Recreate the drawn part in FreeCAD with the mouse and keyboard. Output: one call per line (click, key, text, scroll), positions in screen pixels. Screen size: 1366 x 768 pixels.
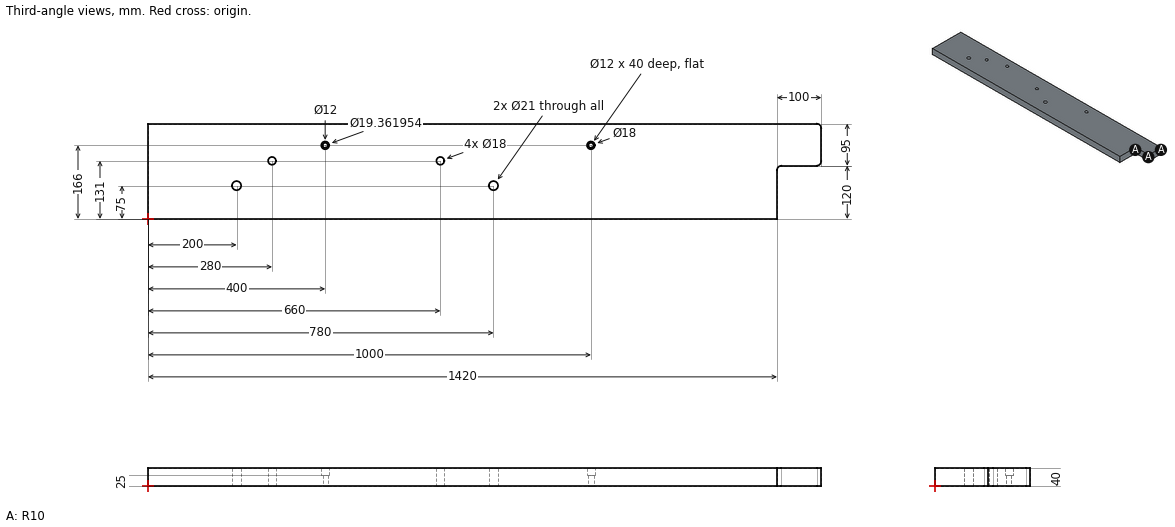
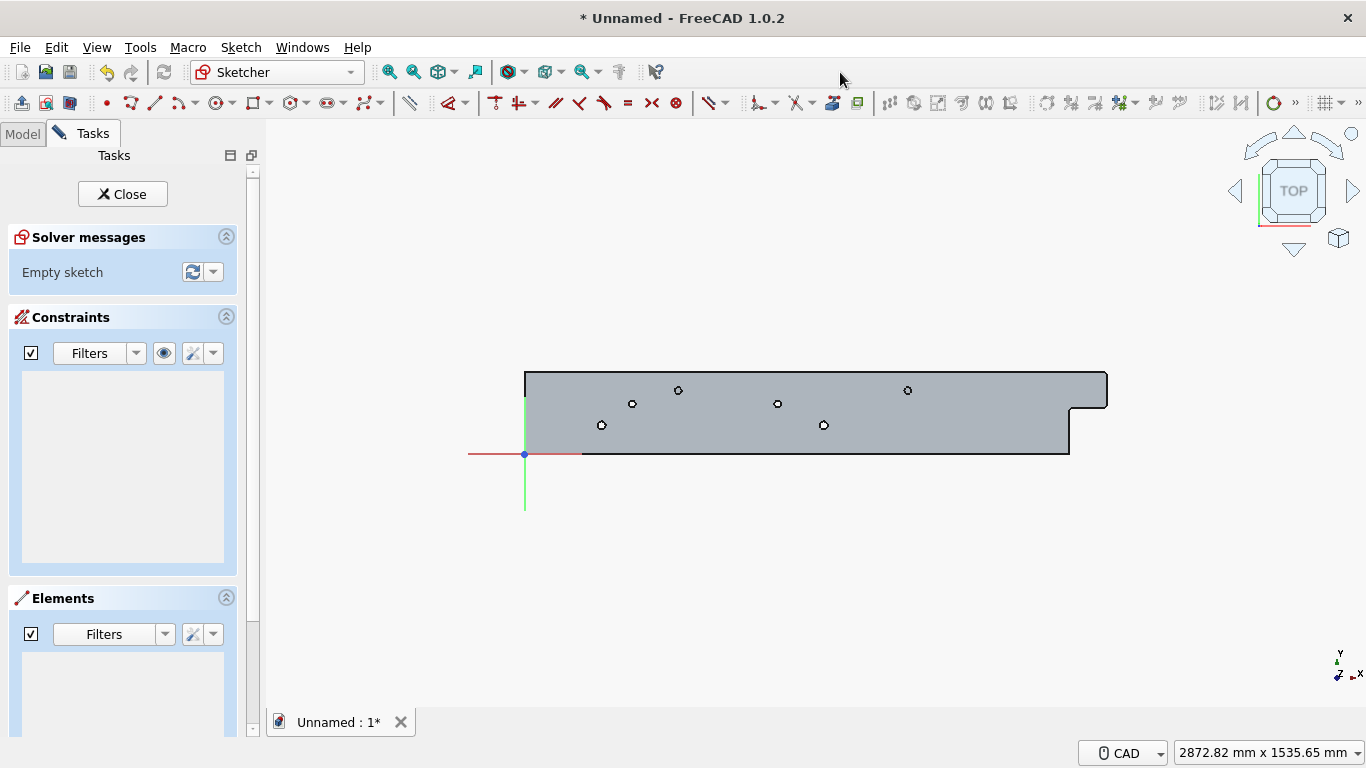
scroll(916, 389, up, 15)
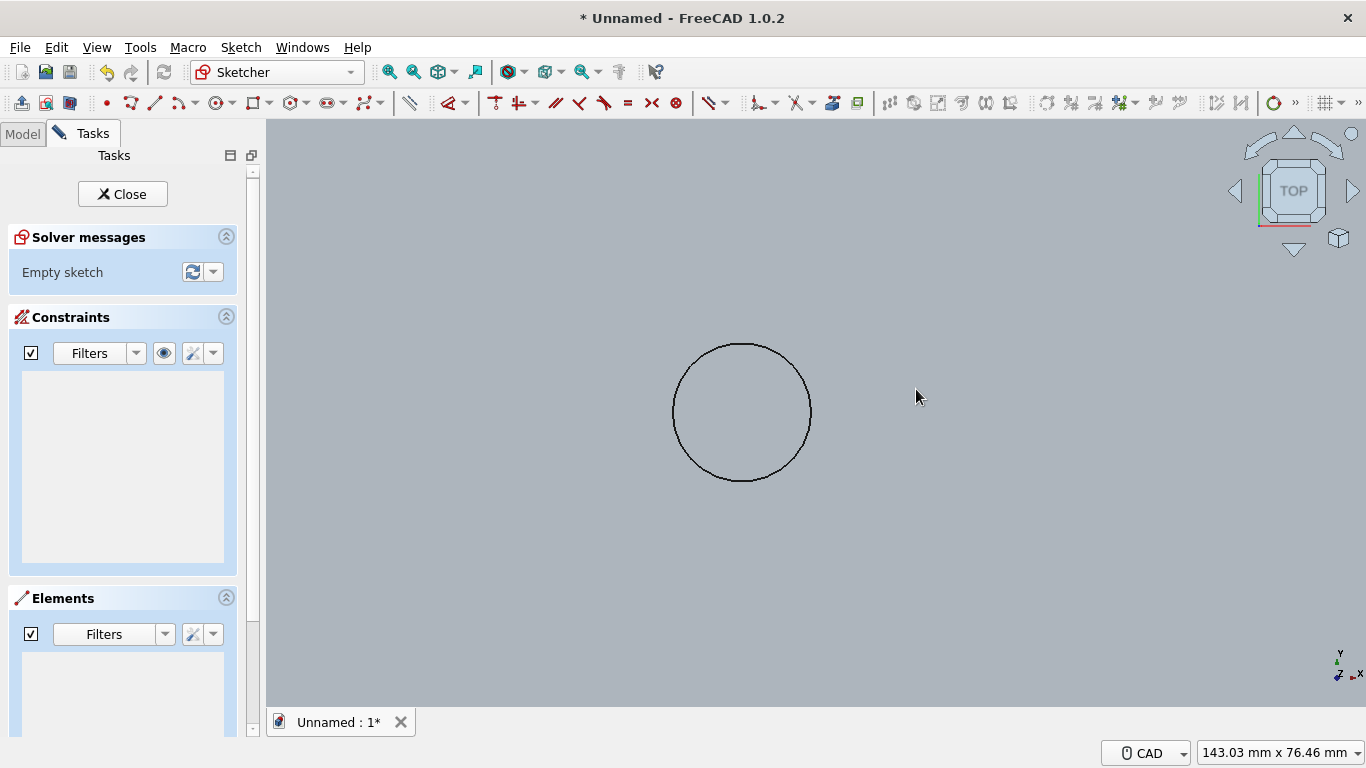
scroll(740, 412, up, 7)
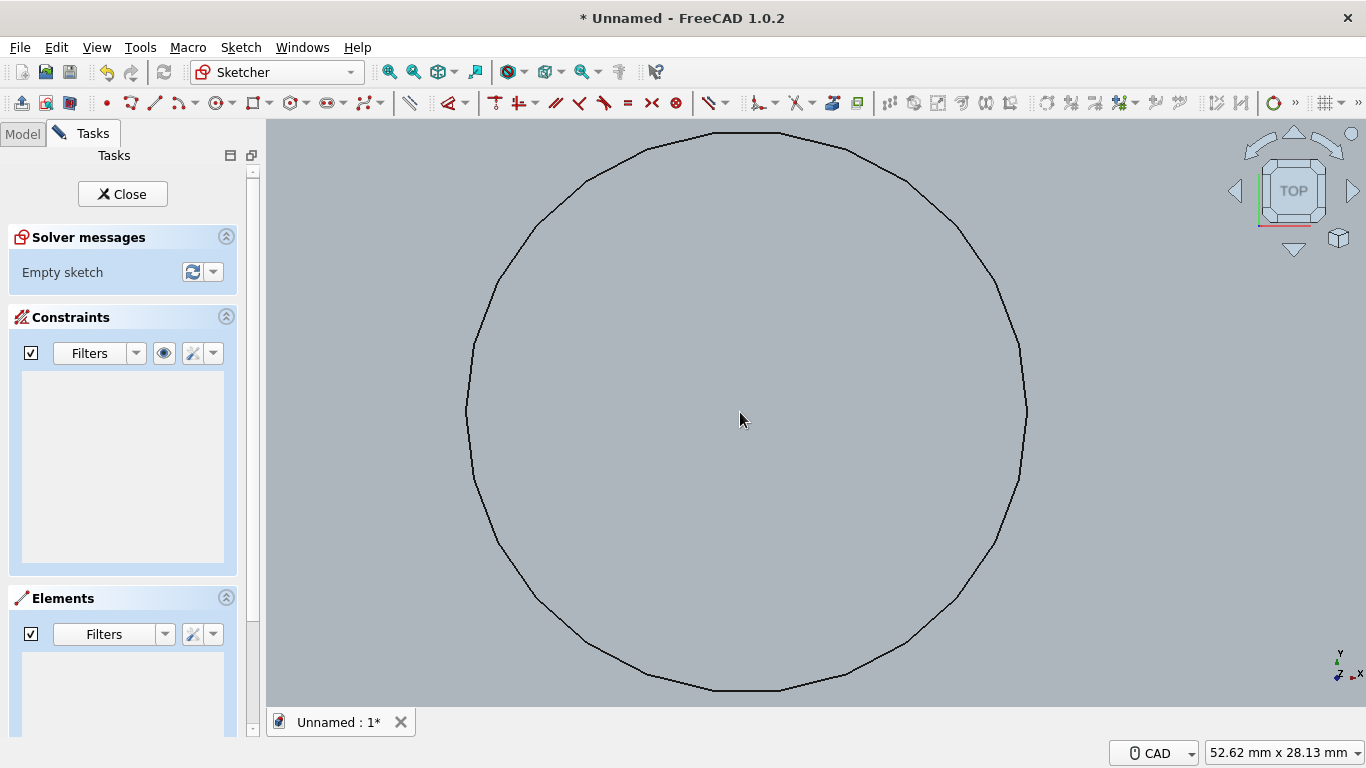
key(g)
key(c)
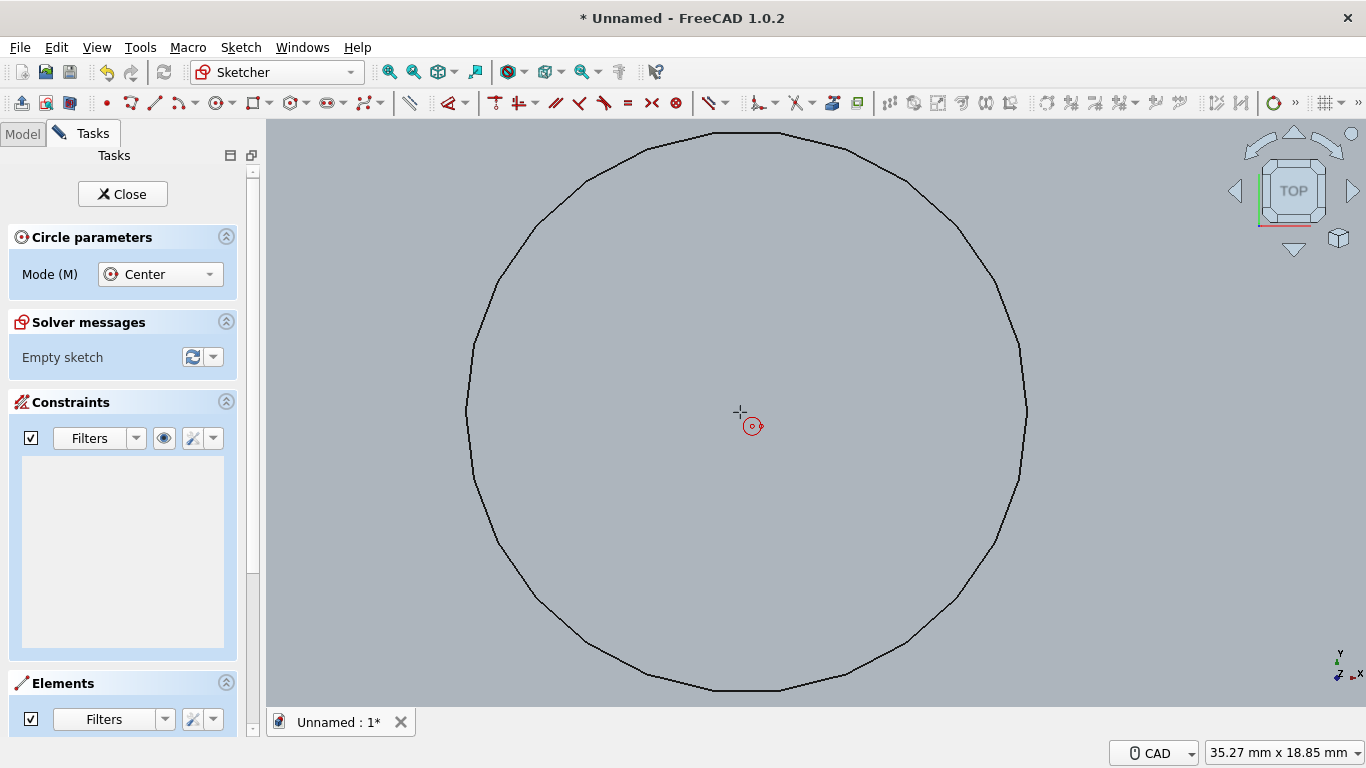
click(747, 412)
click(879, 280)
key(Escape)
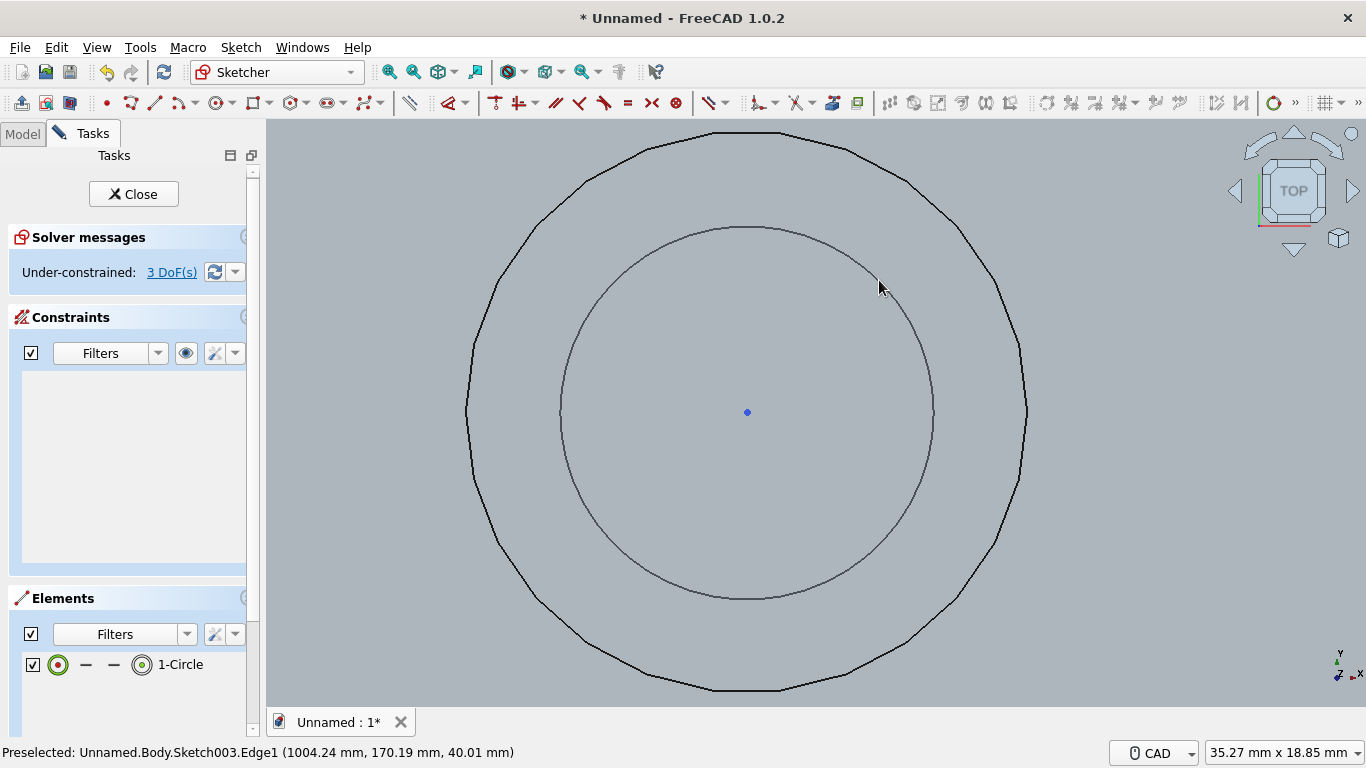
key(d)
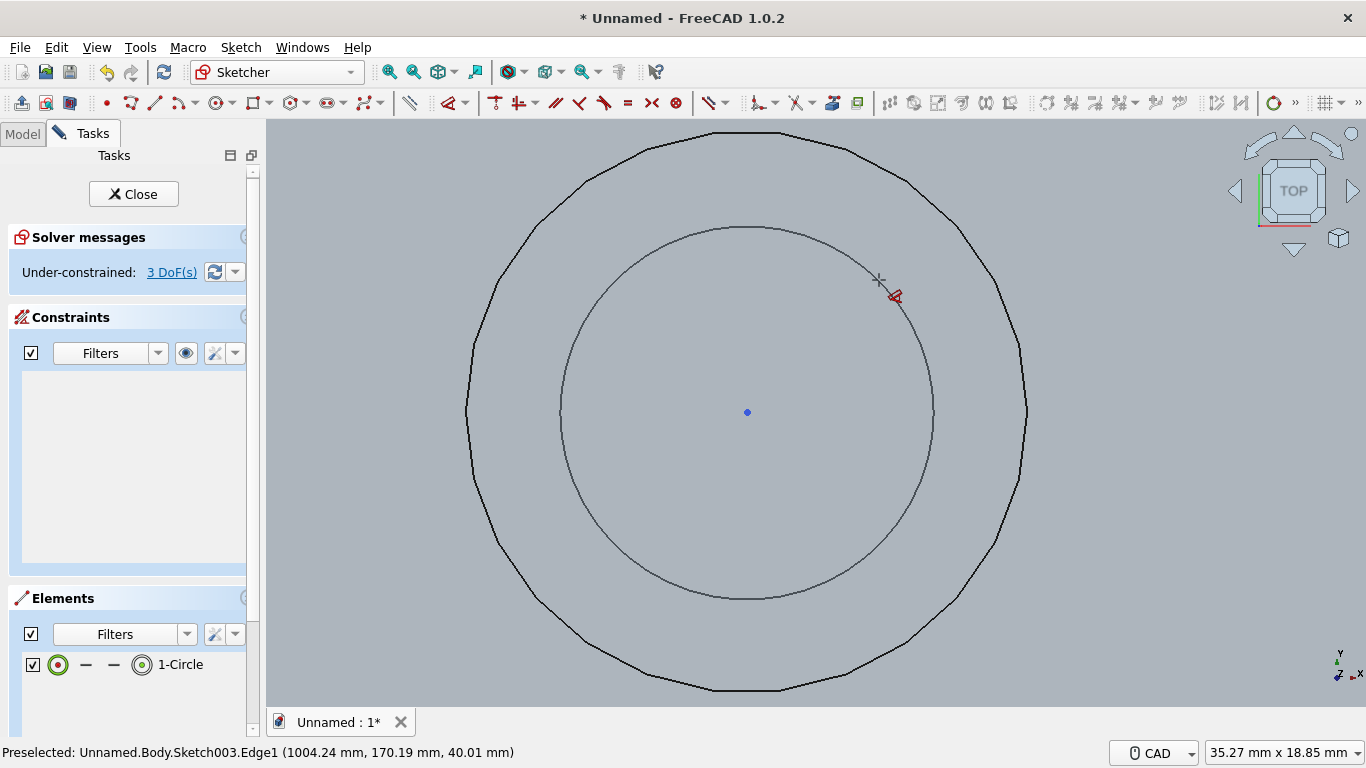
click(879, 281)
click(902, 258)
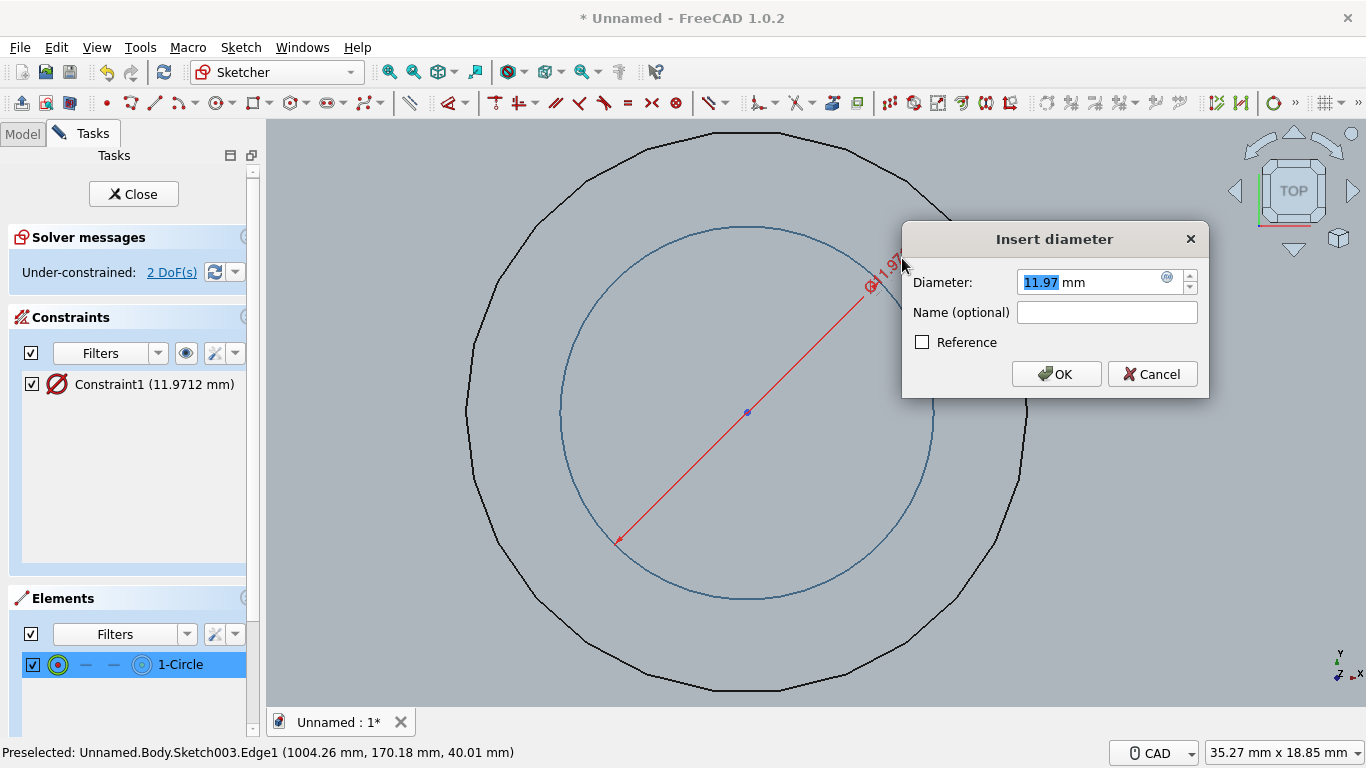
text(12)
key(Return)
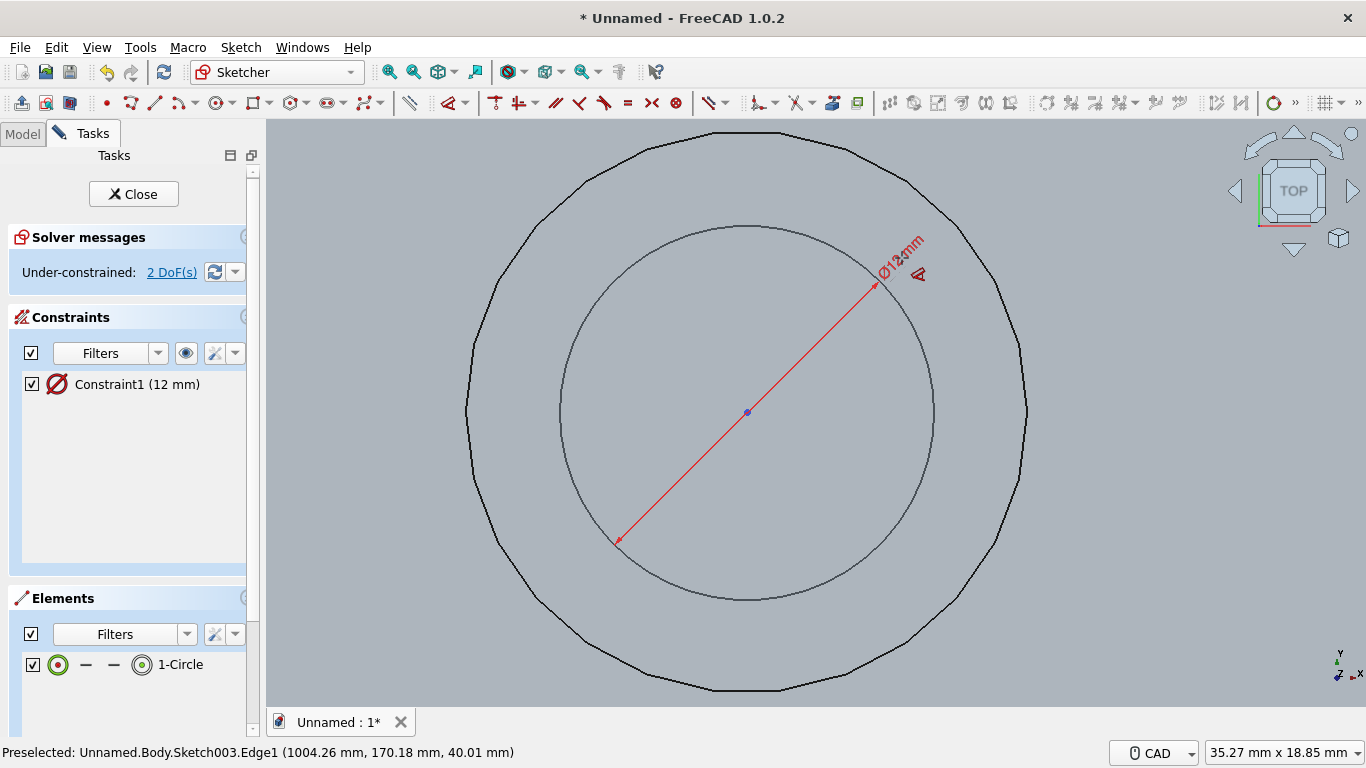
click(747, 413)
click(781, 546)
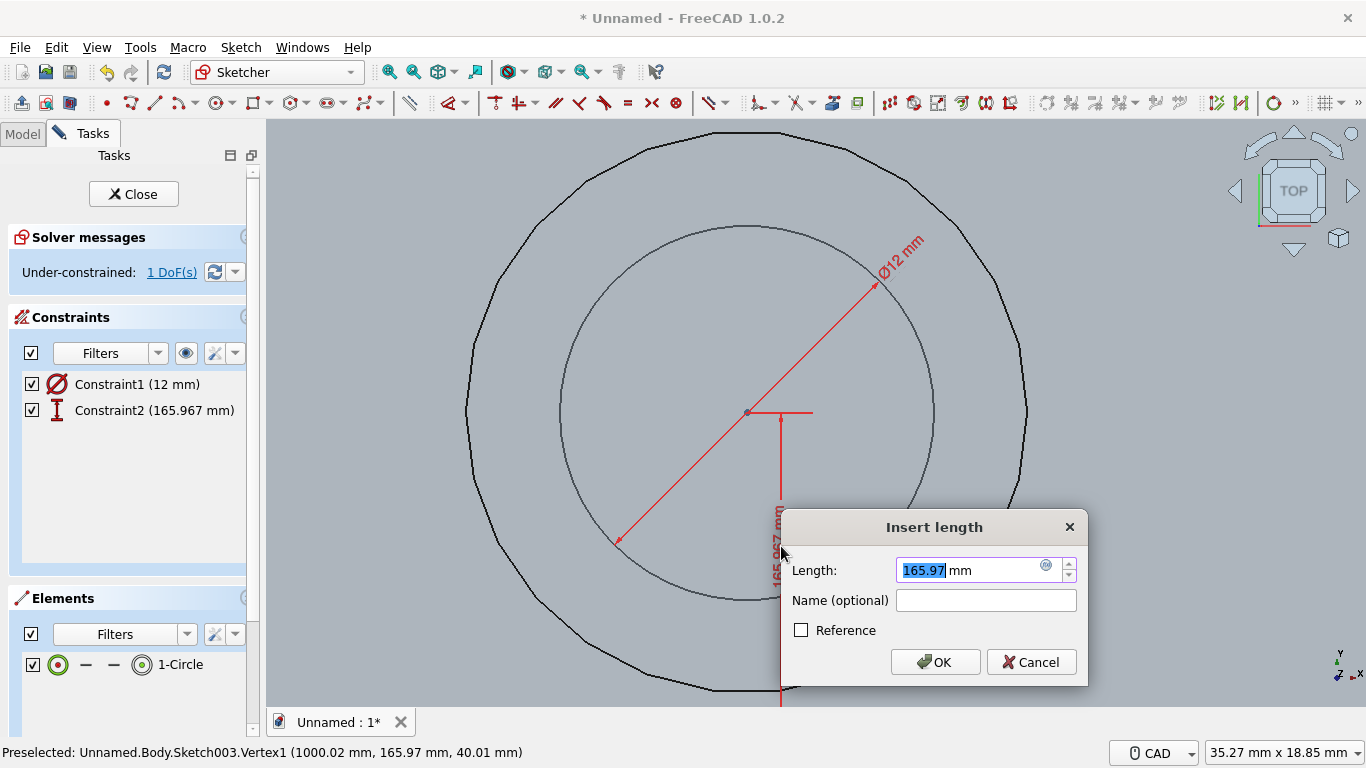
text(166)
key(Return)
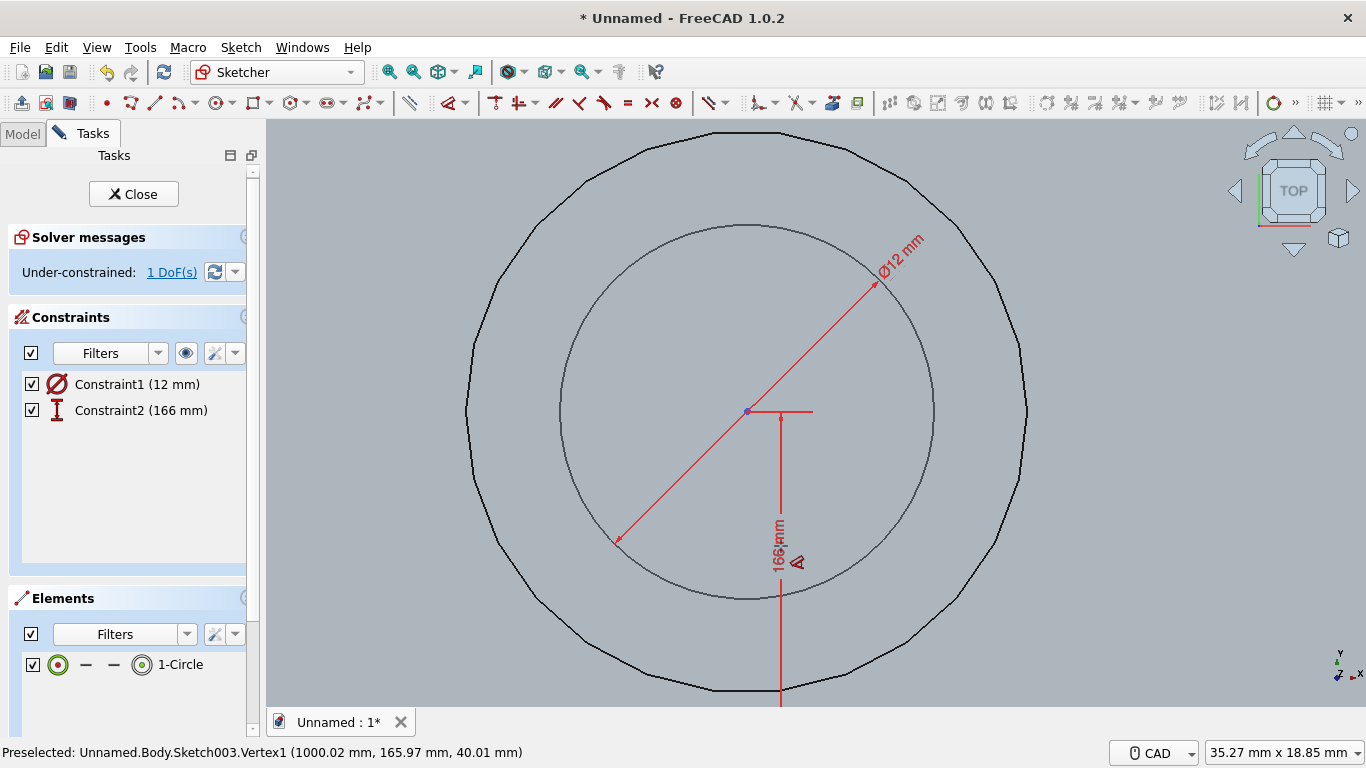
click(747, 412)
click(521, 378)